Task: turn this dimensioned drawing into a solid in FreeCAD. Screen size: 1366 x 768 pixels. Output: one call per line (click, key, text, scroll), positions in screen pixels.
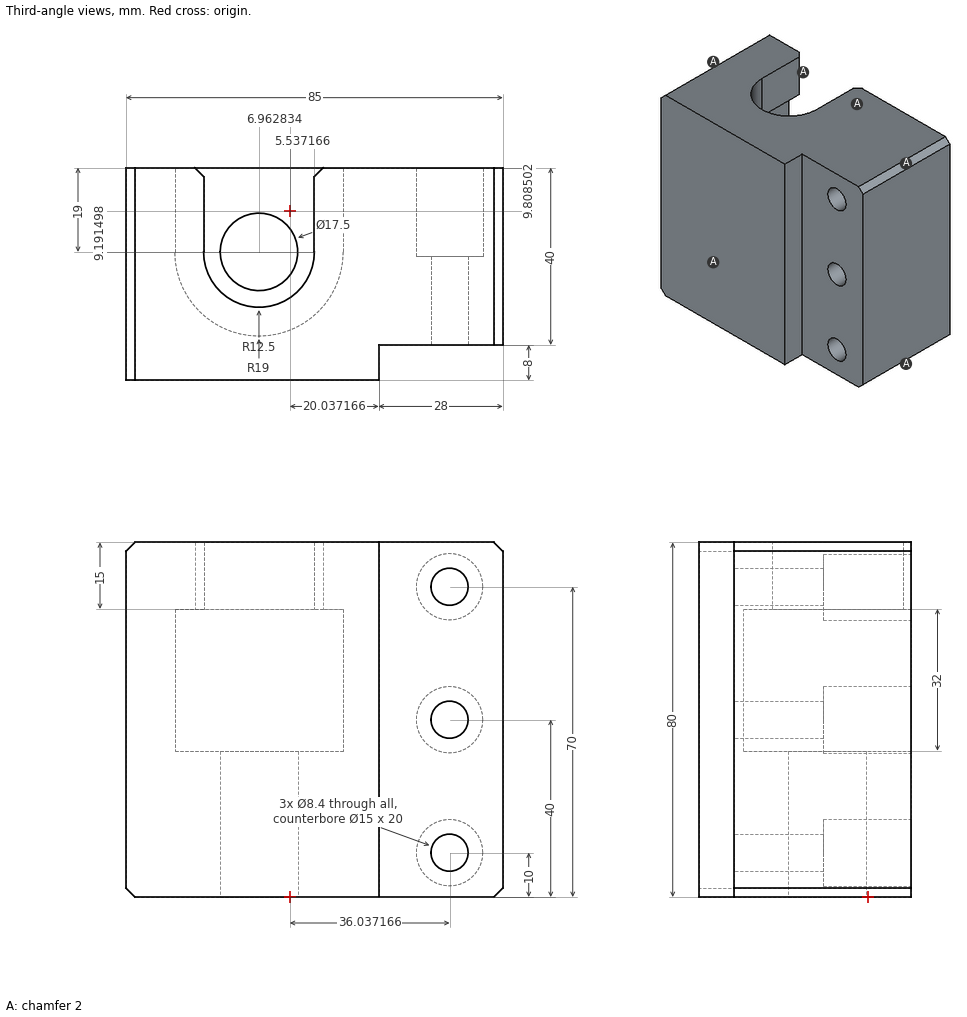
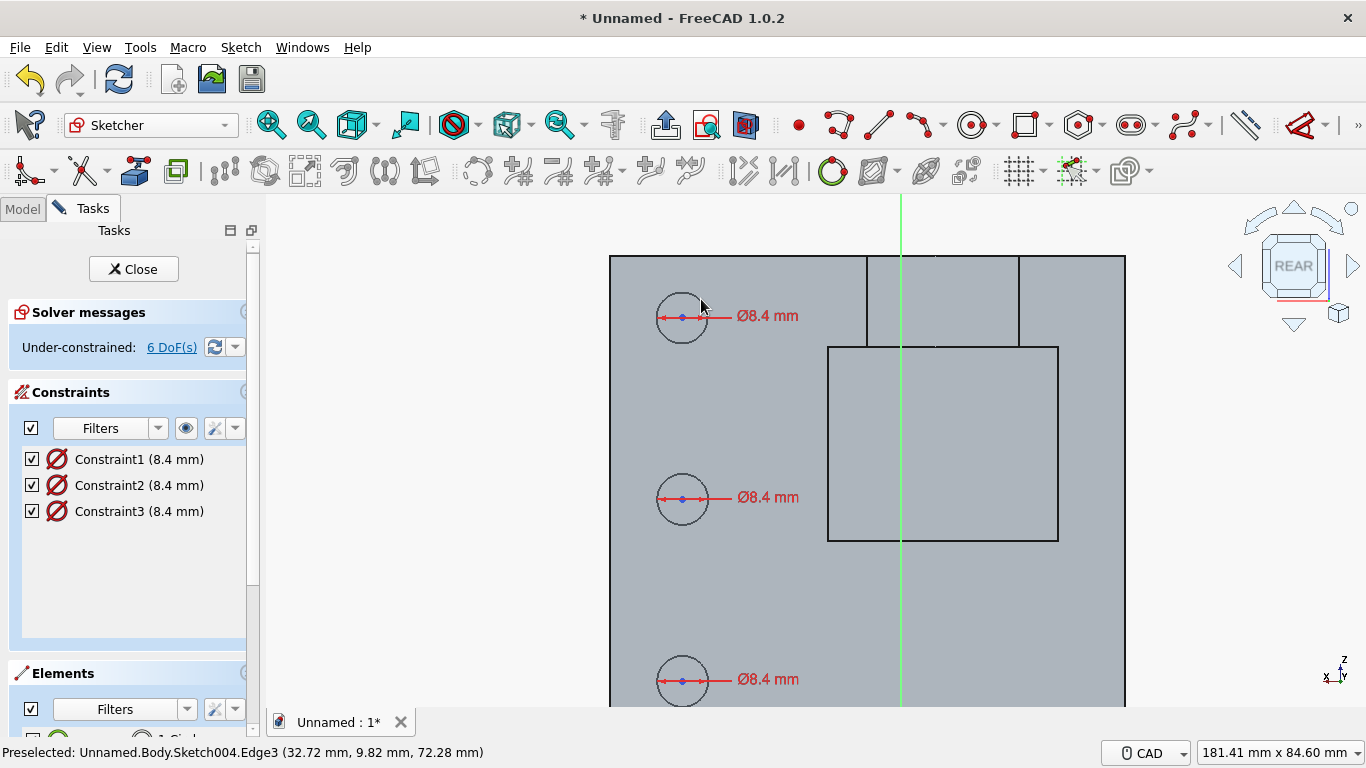
click(1300, 126)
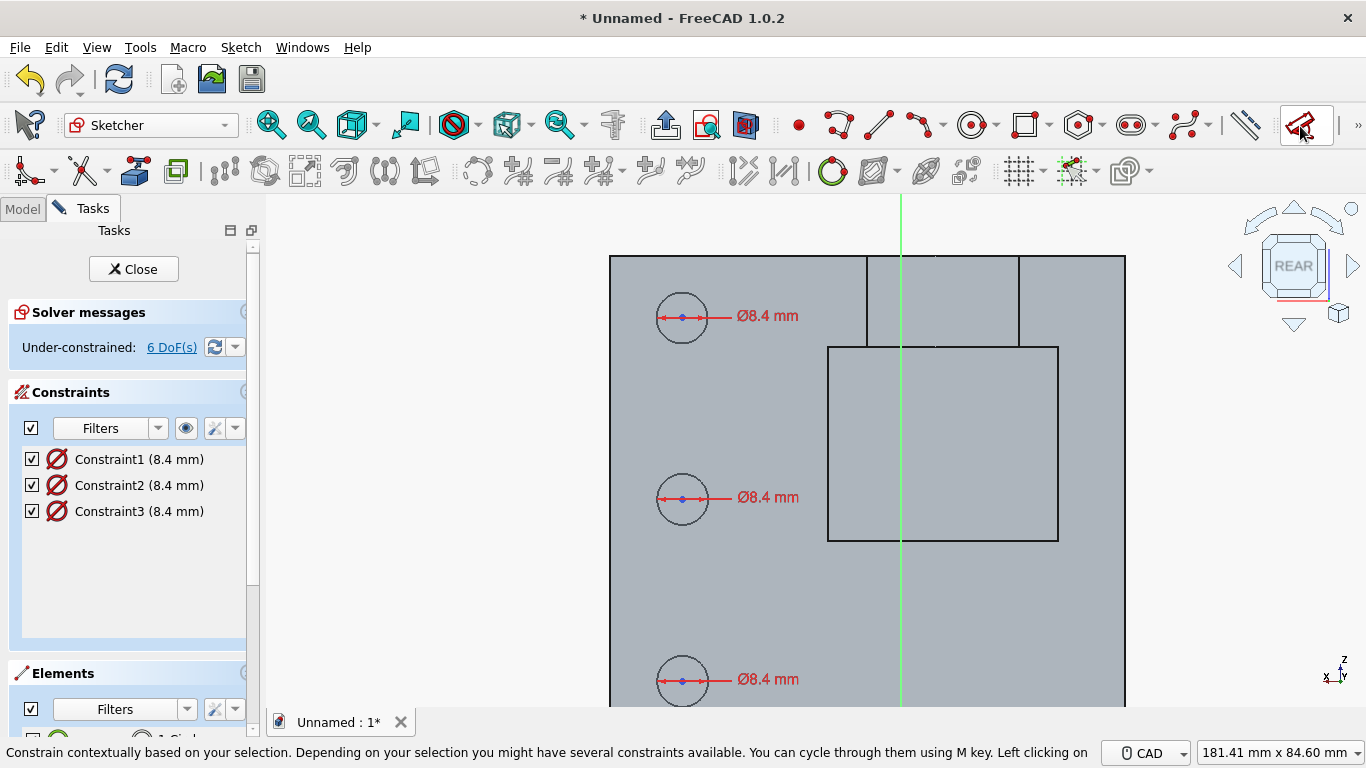
scroll(683, 317, down, 2)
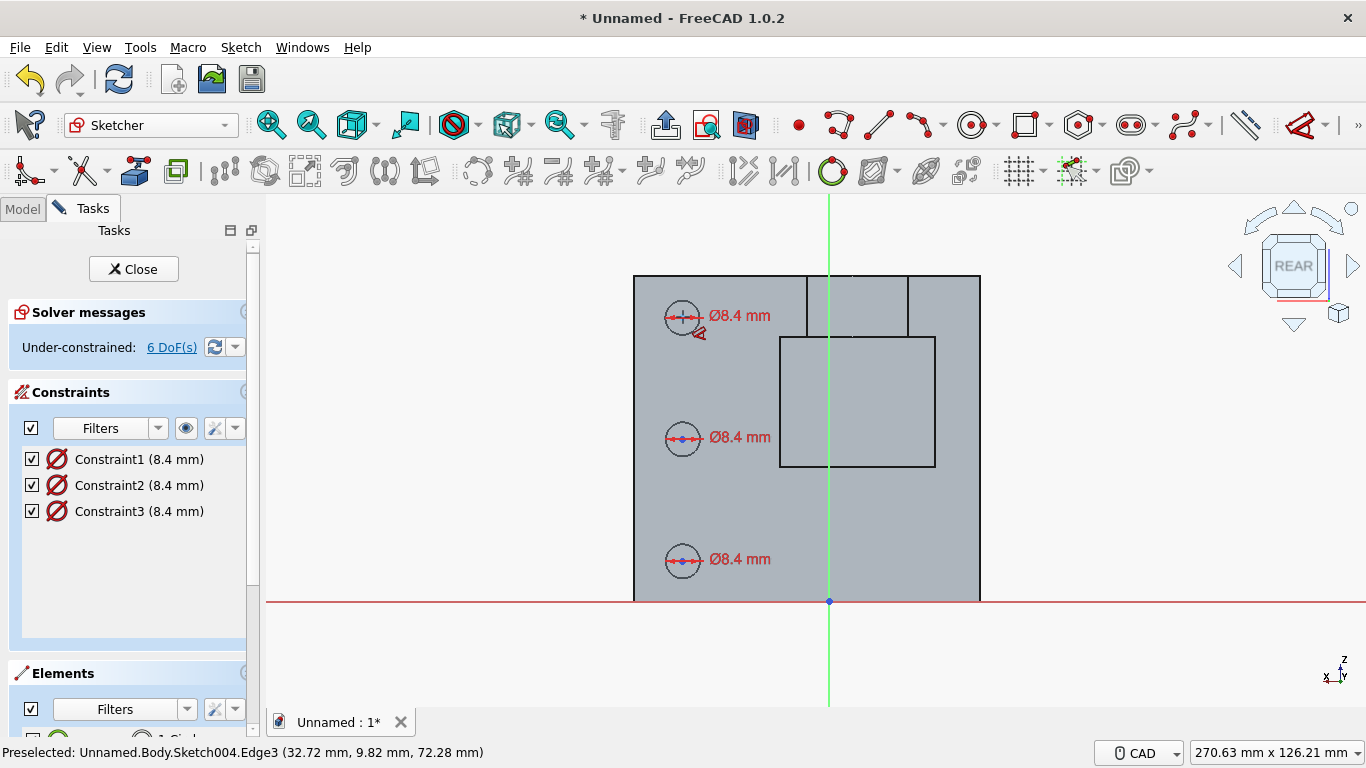
click(683, 561)
click(863, 581)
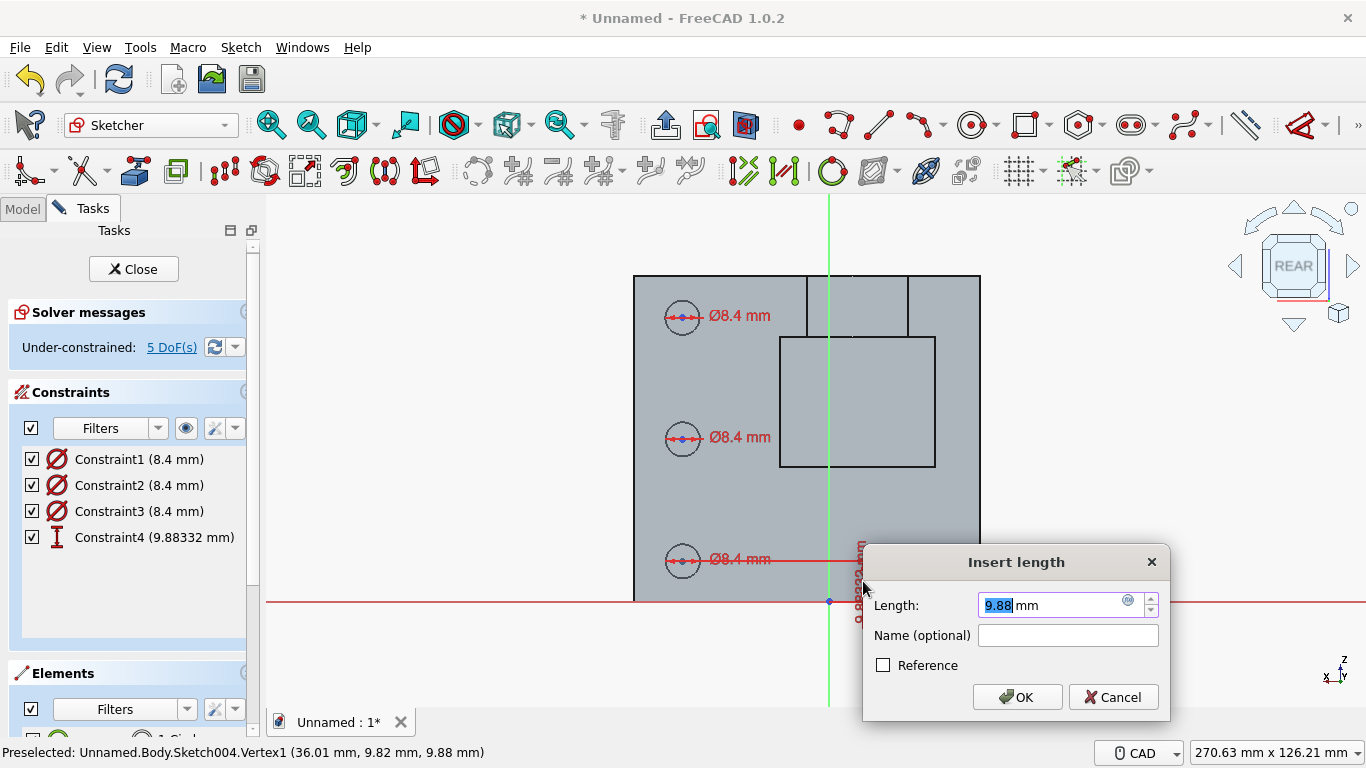
text(10)
key(Return)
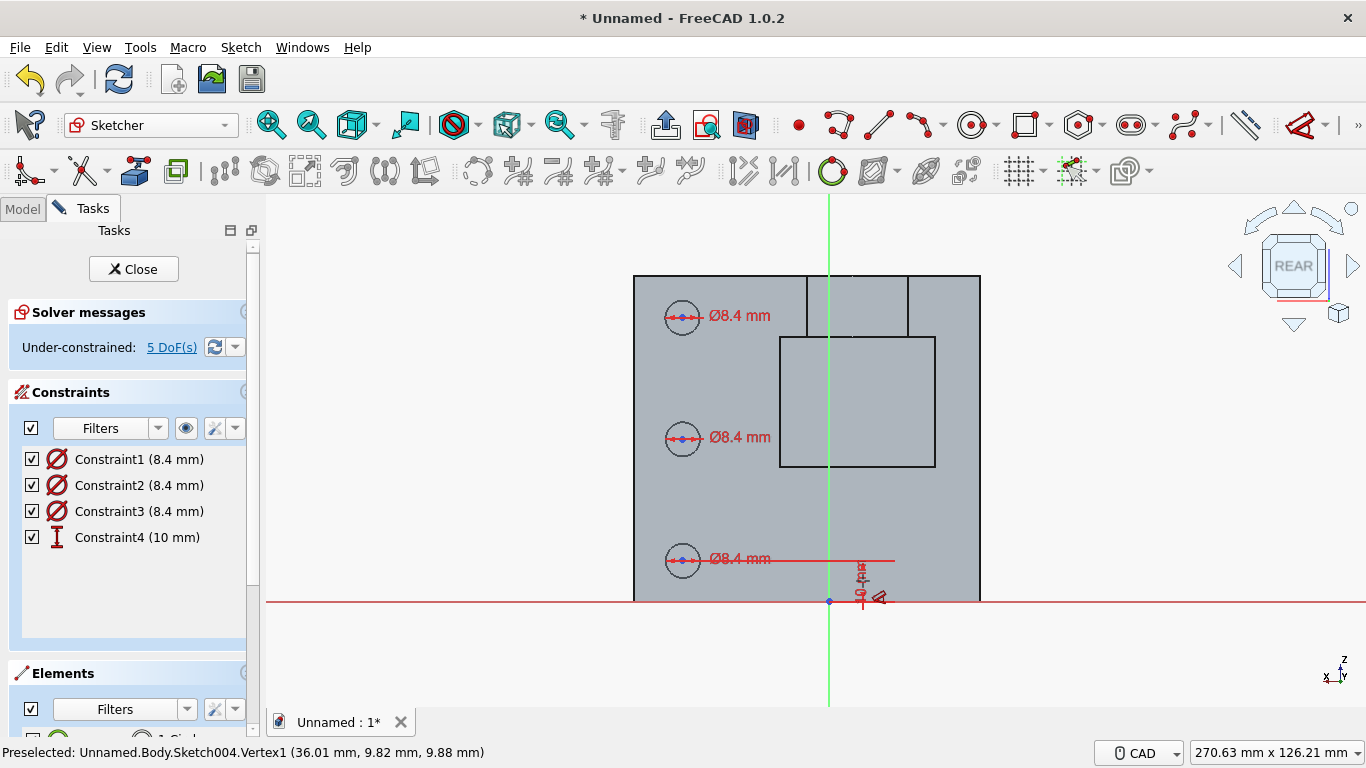
click(683, 439)
click(863, 520)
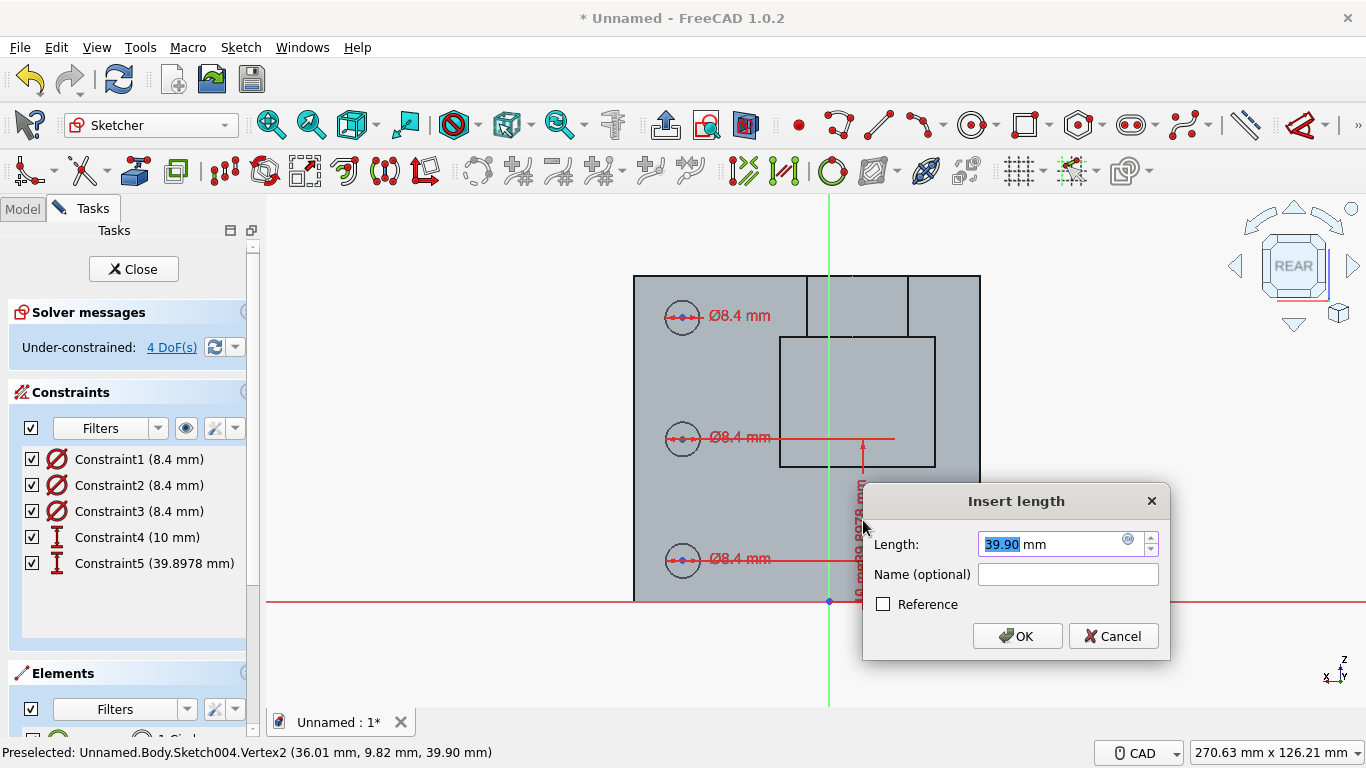
text(40)
key(Return)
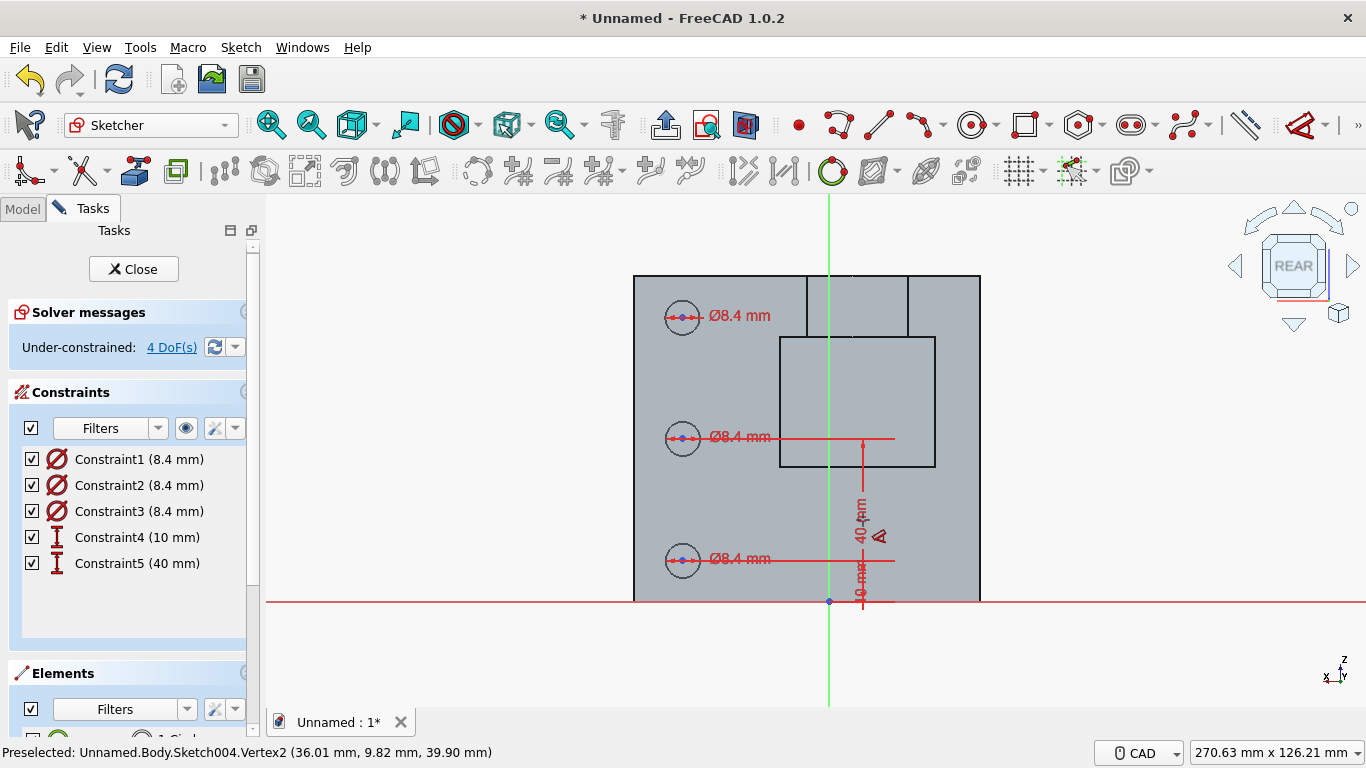
click(682, 318)
click(863, 460)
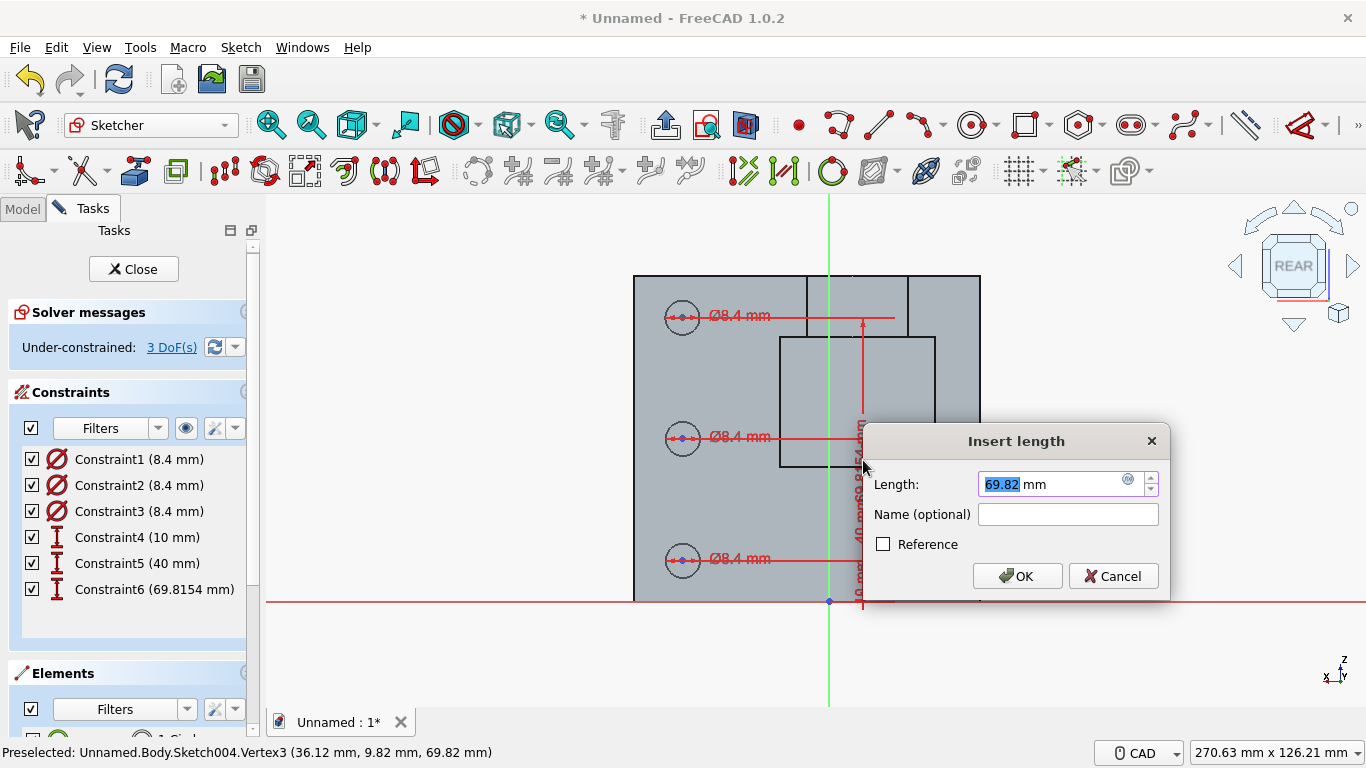
text(70)
key(Return)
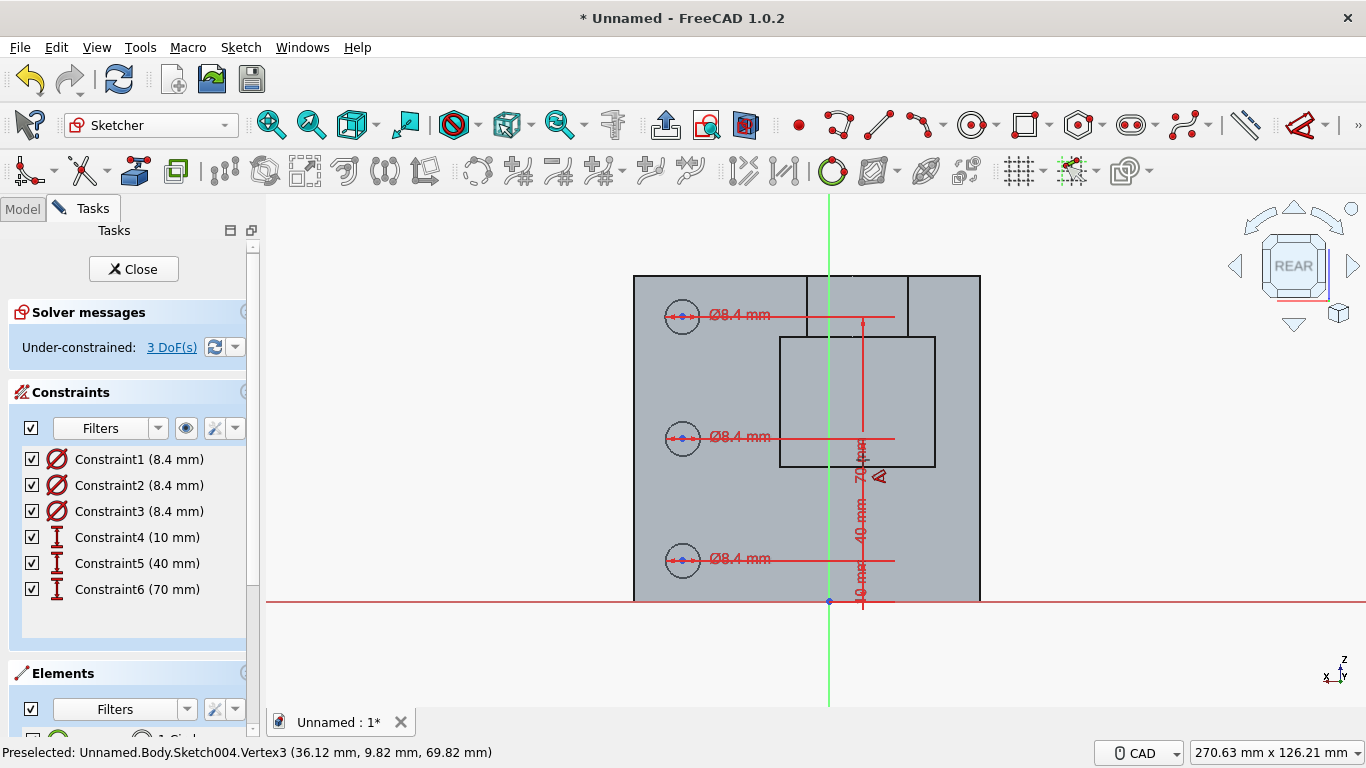
click(683, 561)
click(756, 636)